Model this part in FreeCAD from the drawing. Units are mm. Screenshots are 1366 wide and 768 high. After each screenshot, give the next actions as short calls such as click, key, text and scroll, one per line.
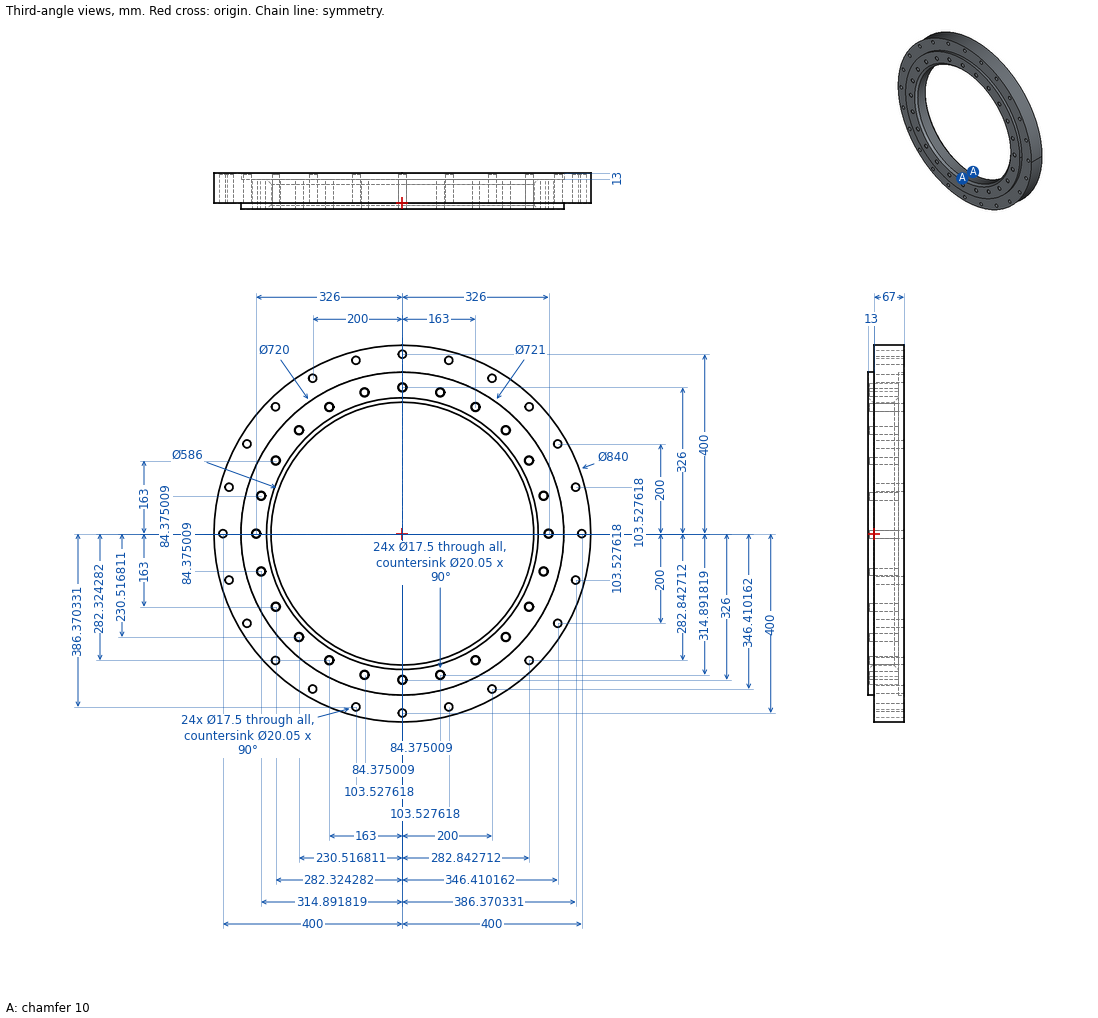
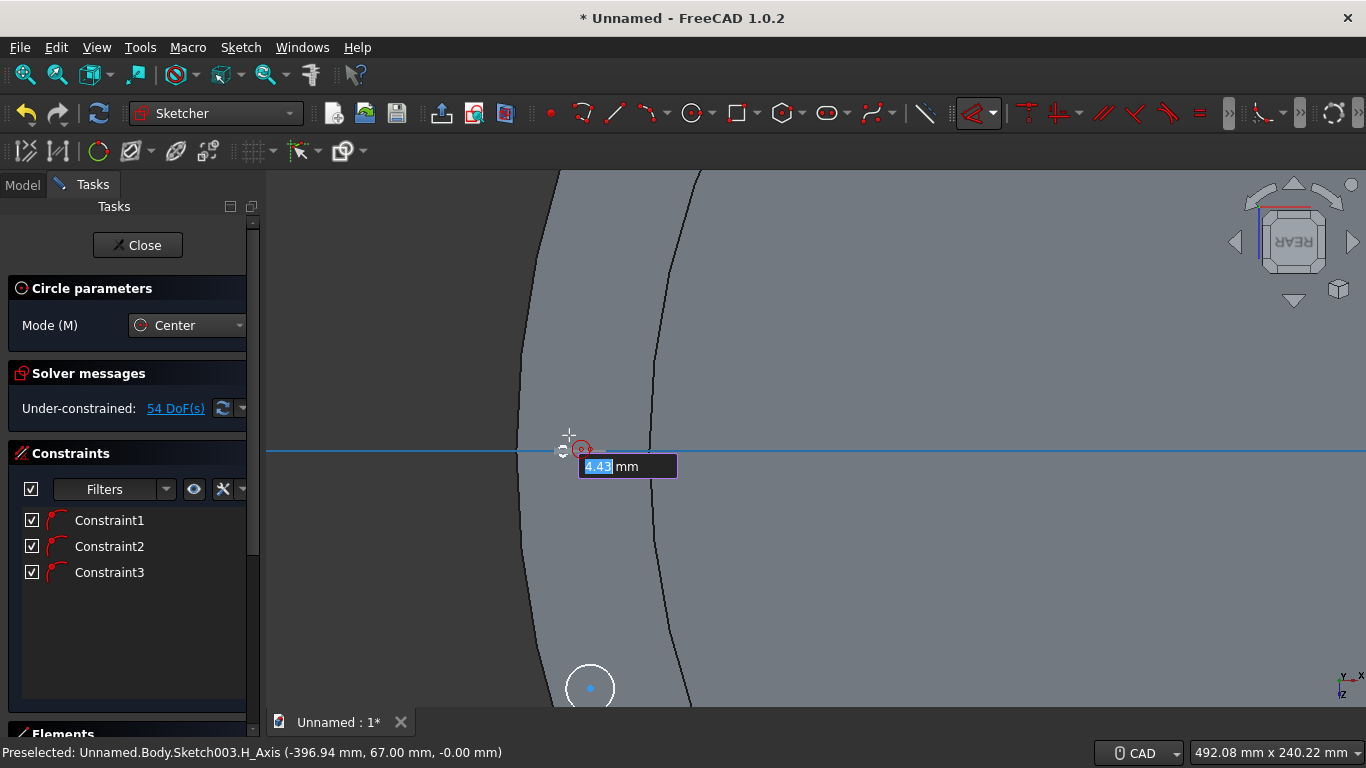
click(568, 433)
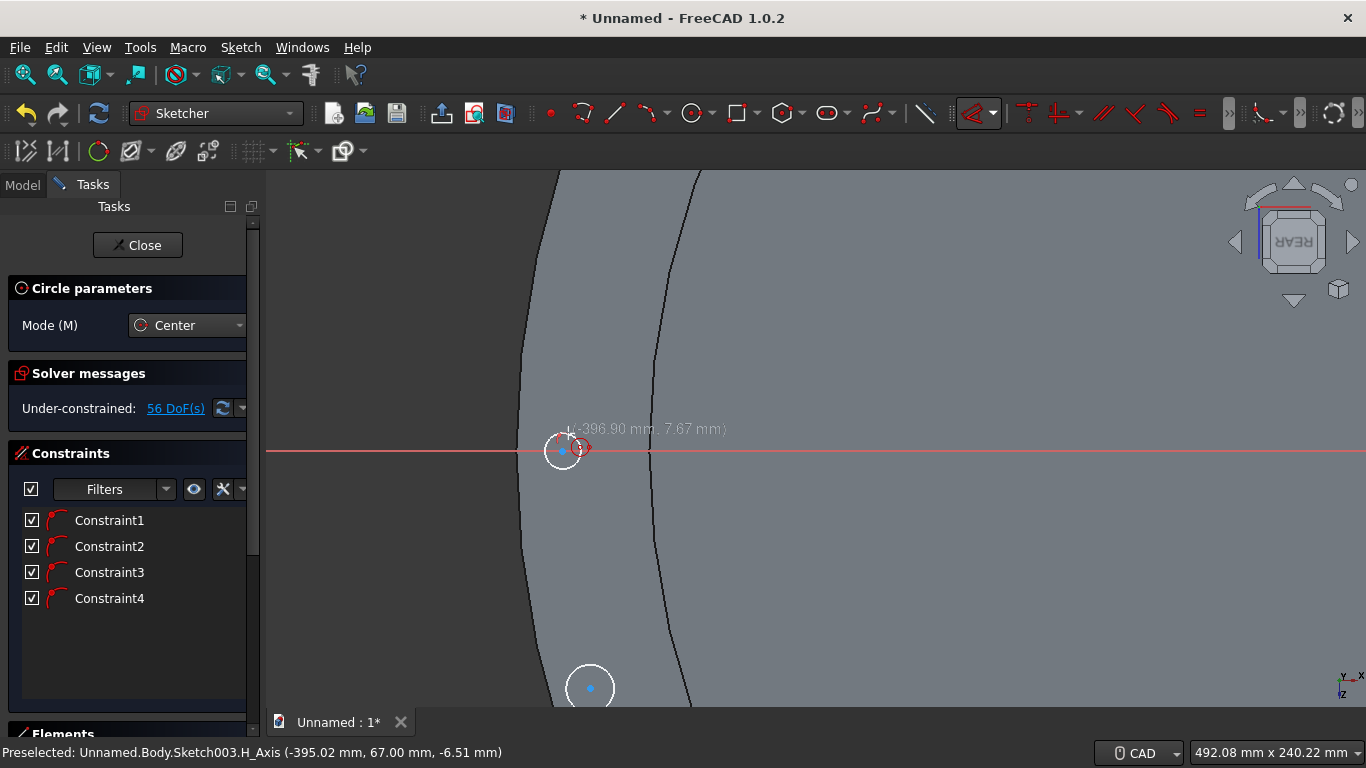
scroll(568, 435, down, 8)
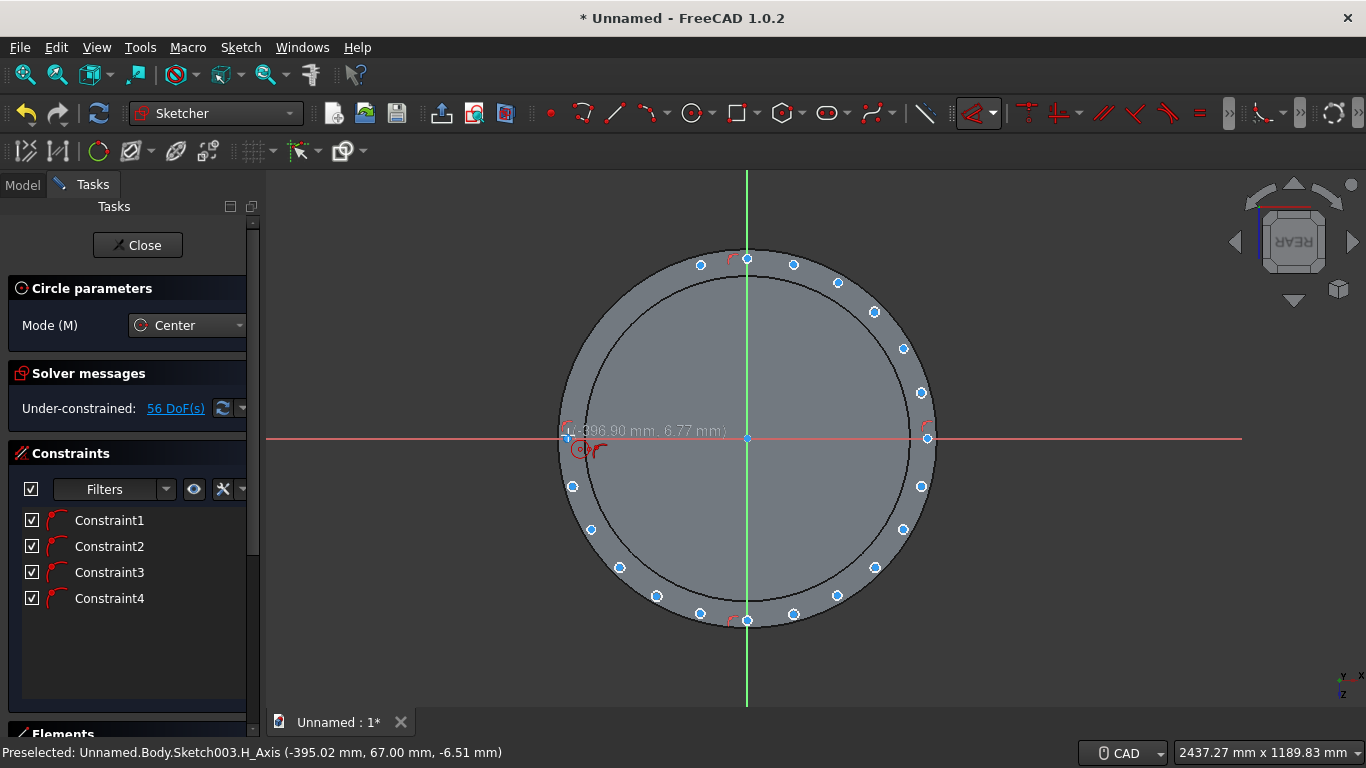
click(573, 392)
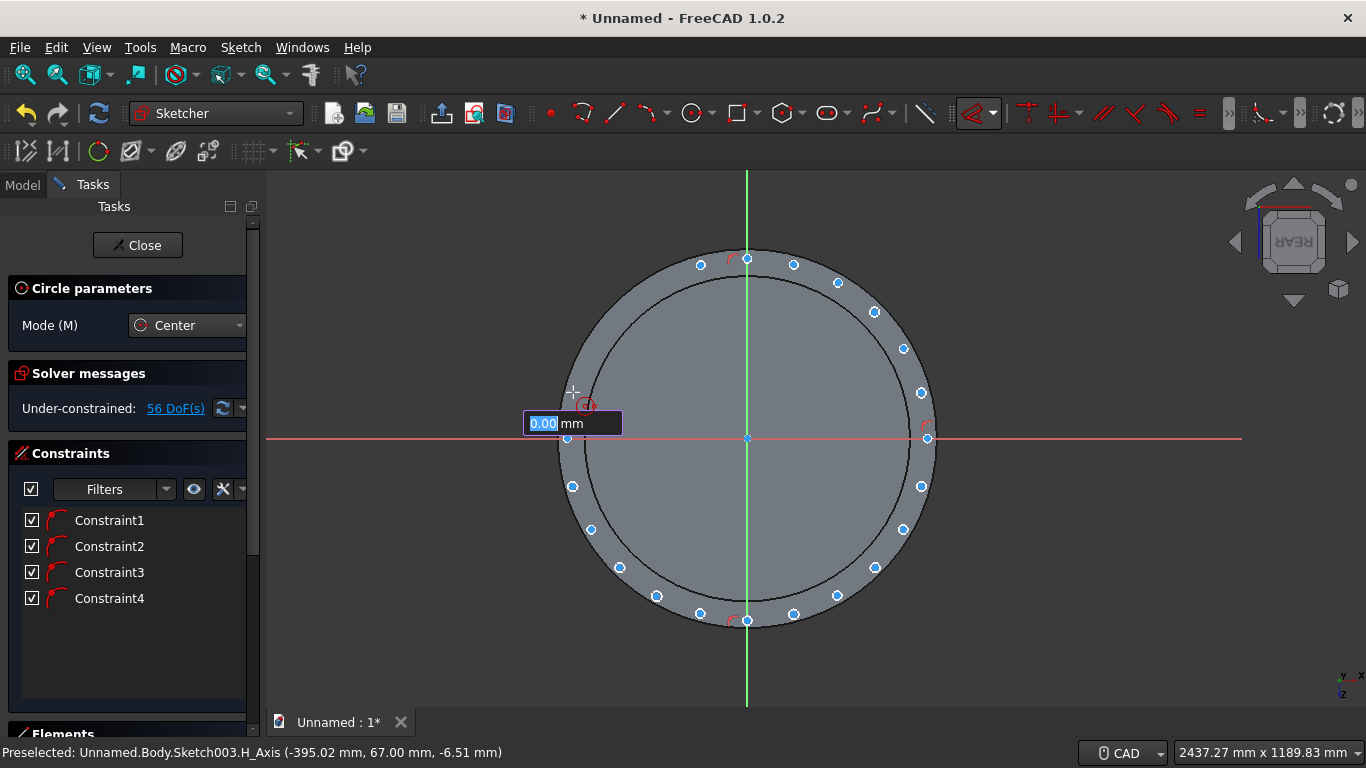
scroll(576, 389, up, 7)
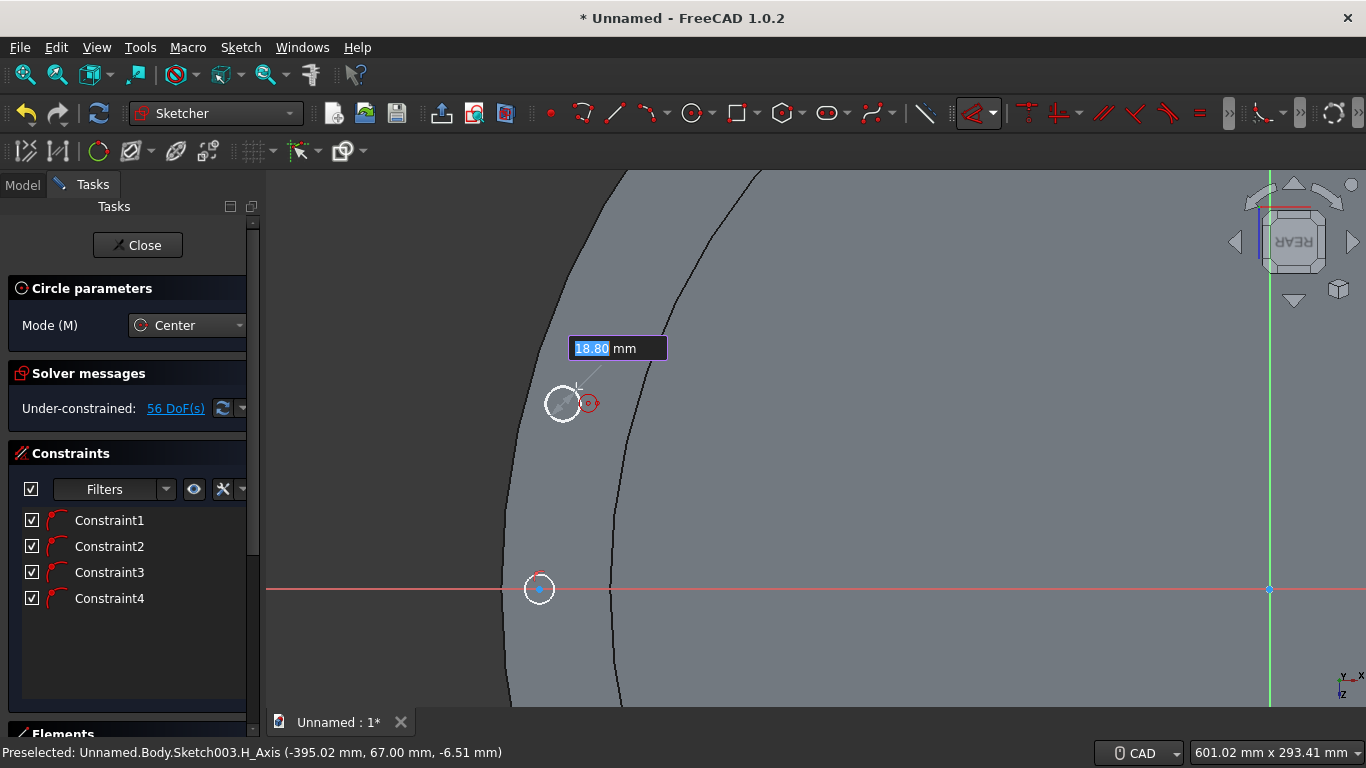
click(574, 388)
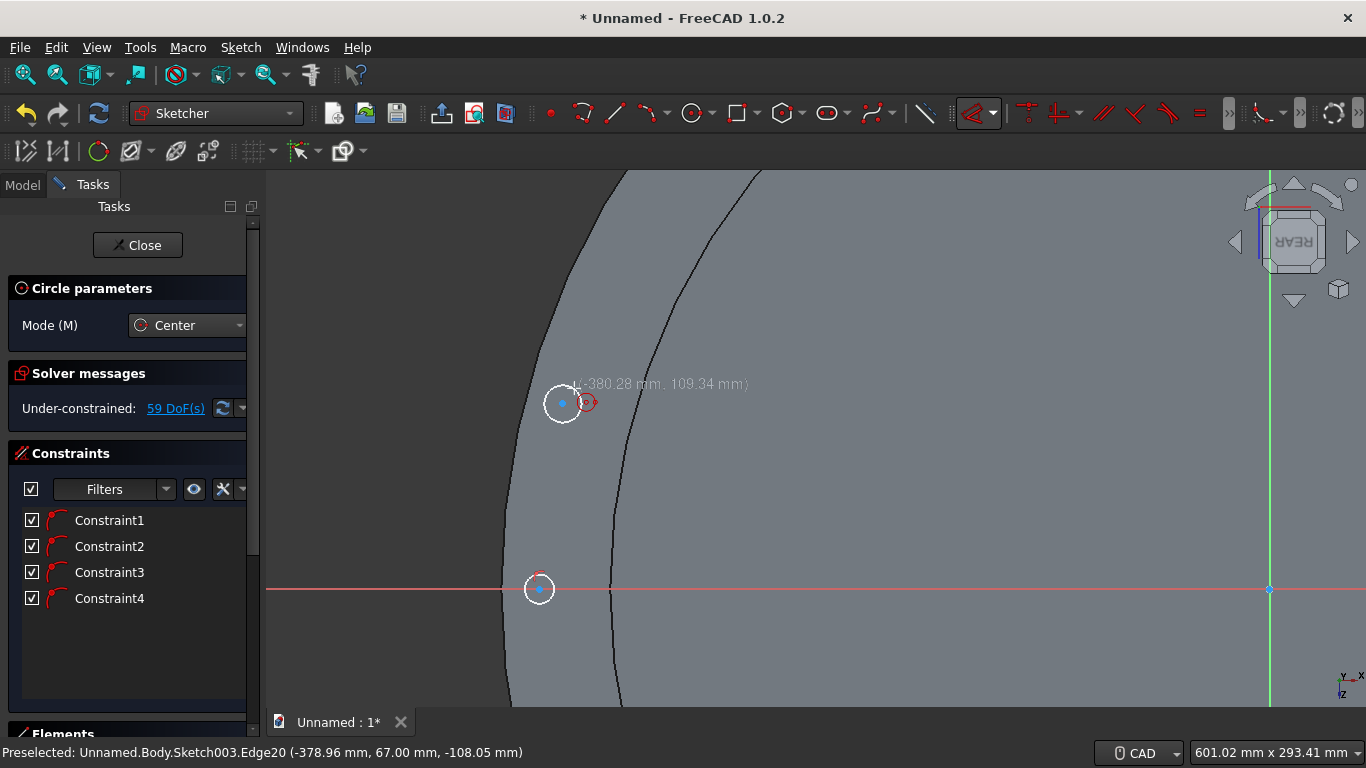
scroll(636, 223, up, 2)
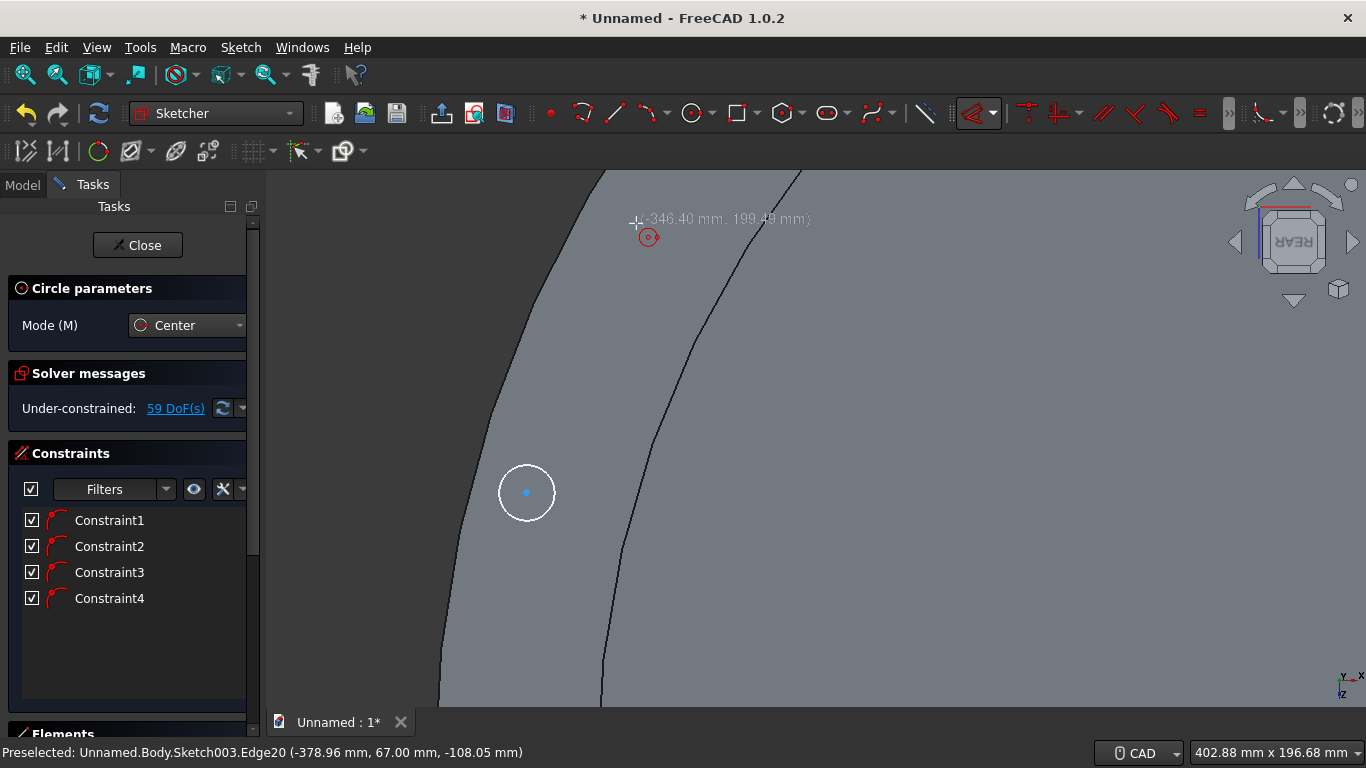
scroll(582, 373, down, 9)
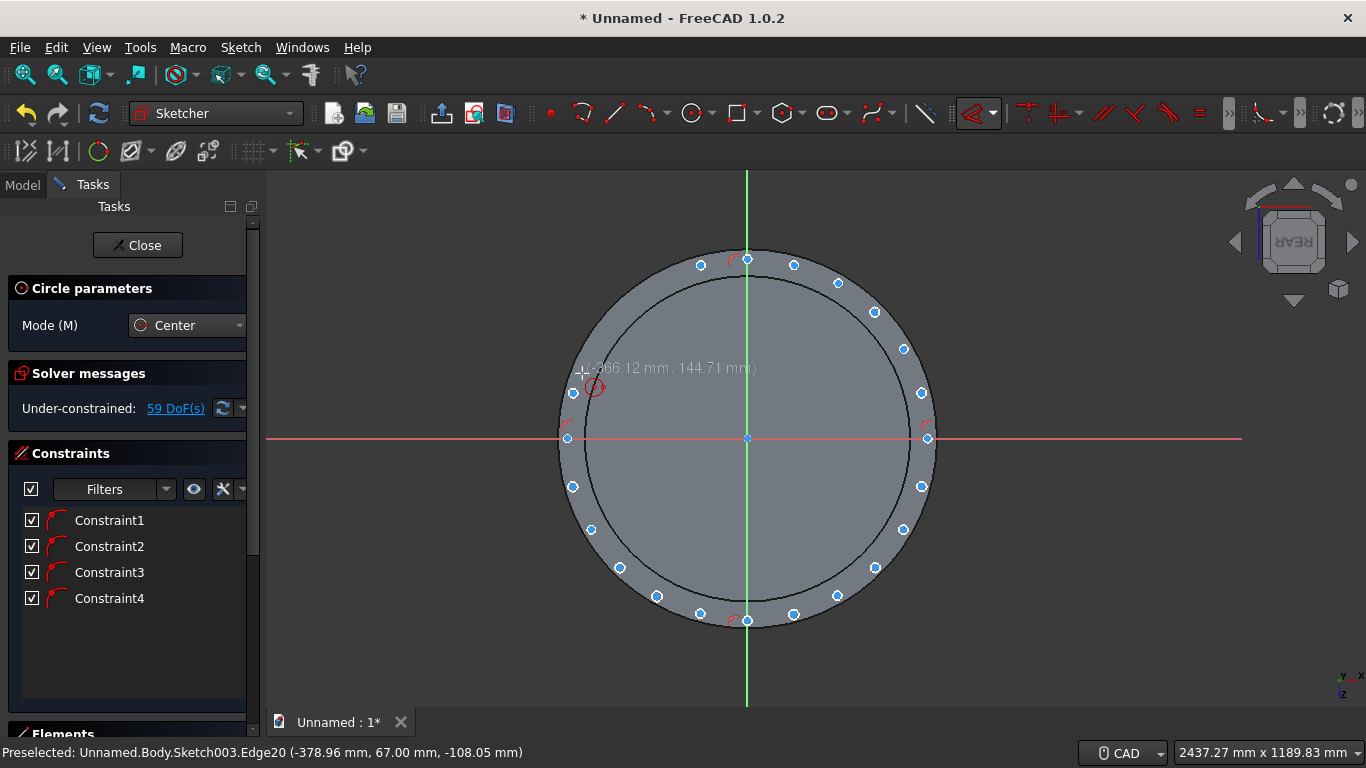
click(591, 349)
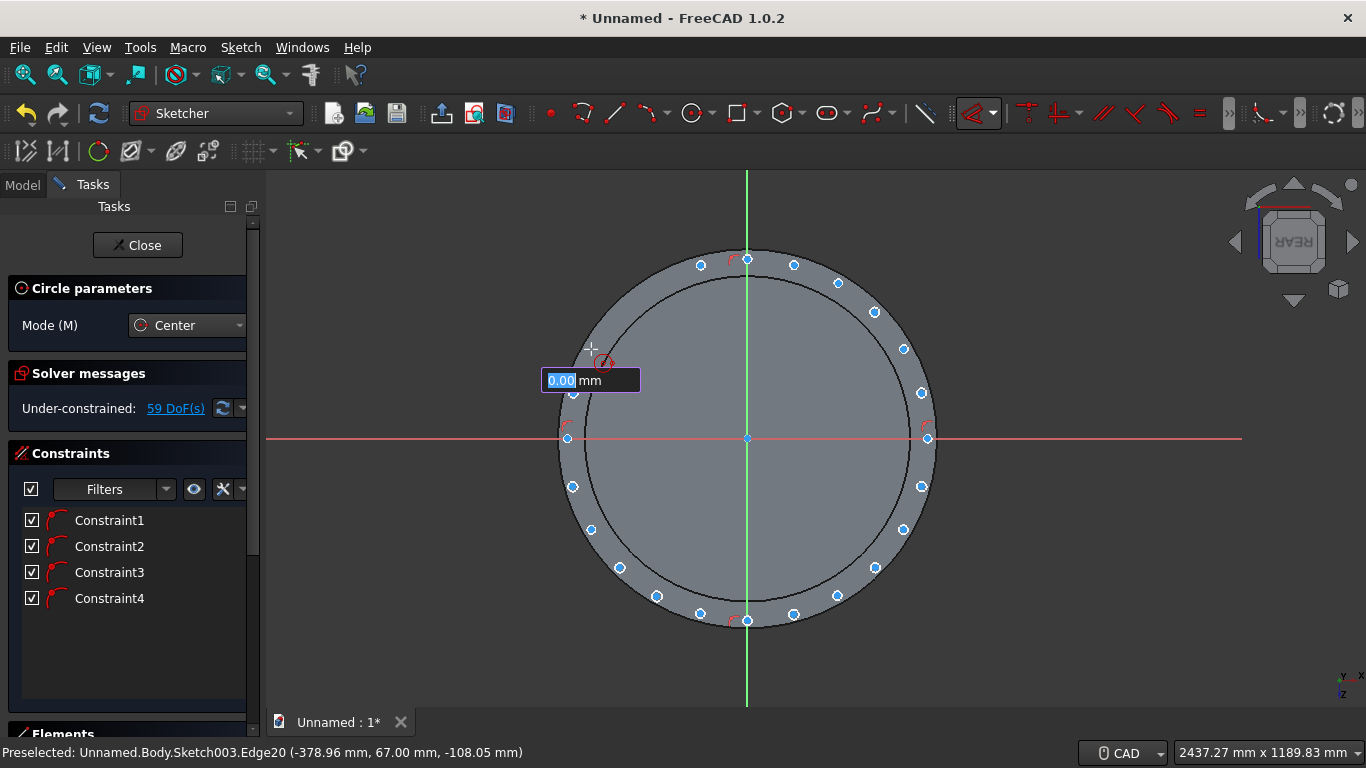
scroll(594, 346, up, 7)